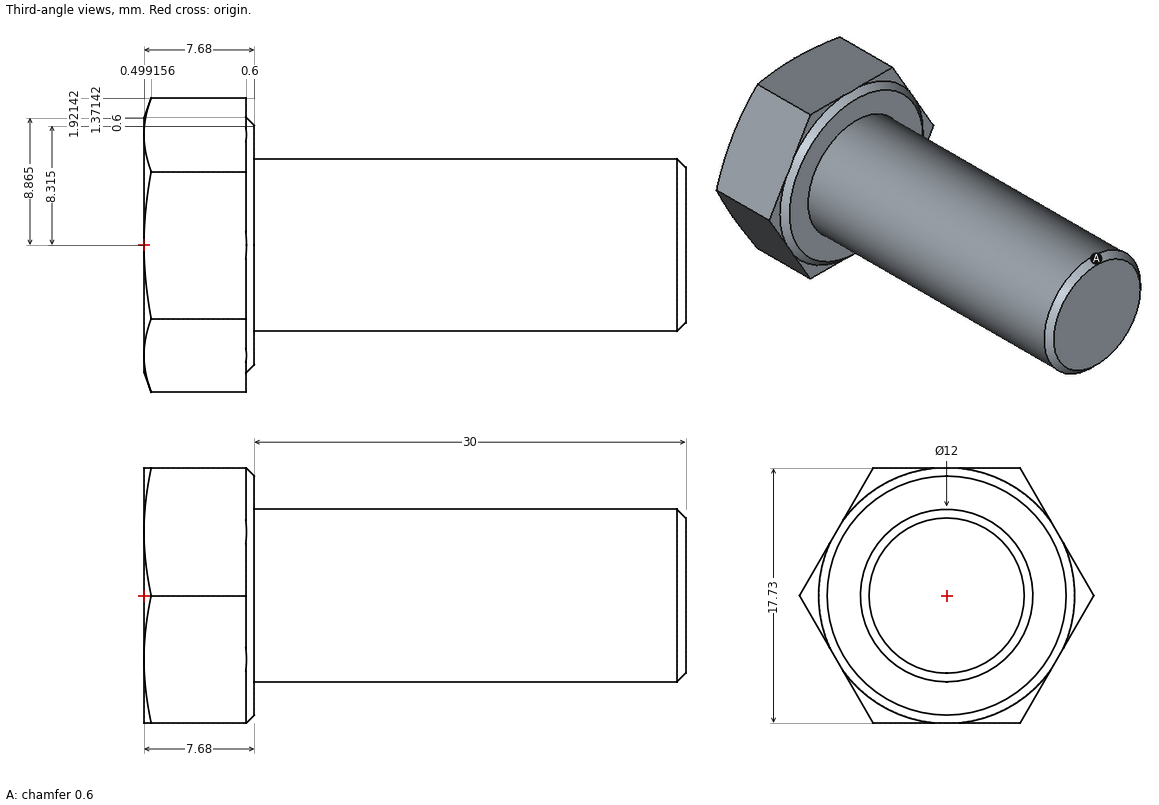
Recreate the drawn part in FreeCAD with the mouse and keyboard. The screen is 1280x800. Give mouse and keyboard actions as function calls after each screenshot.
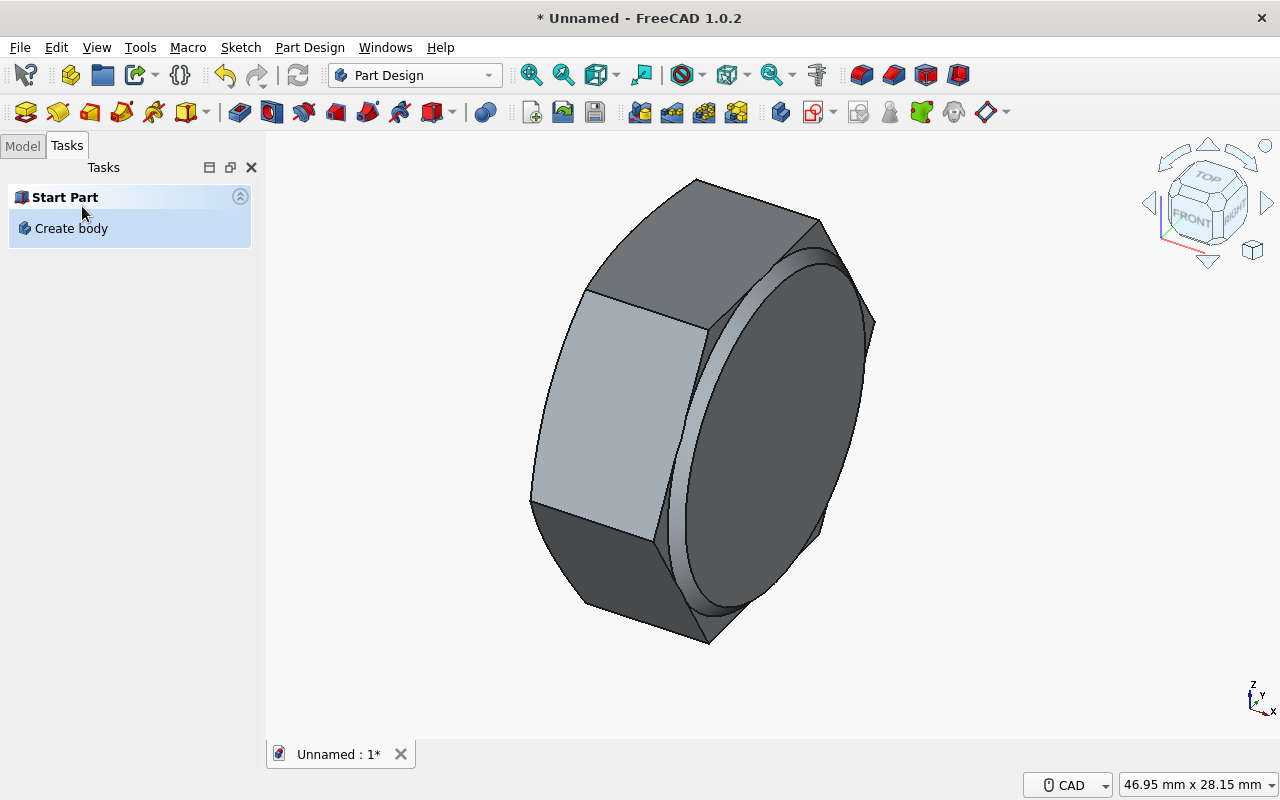
click(532, 76)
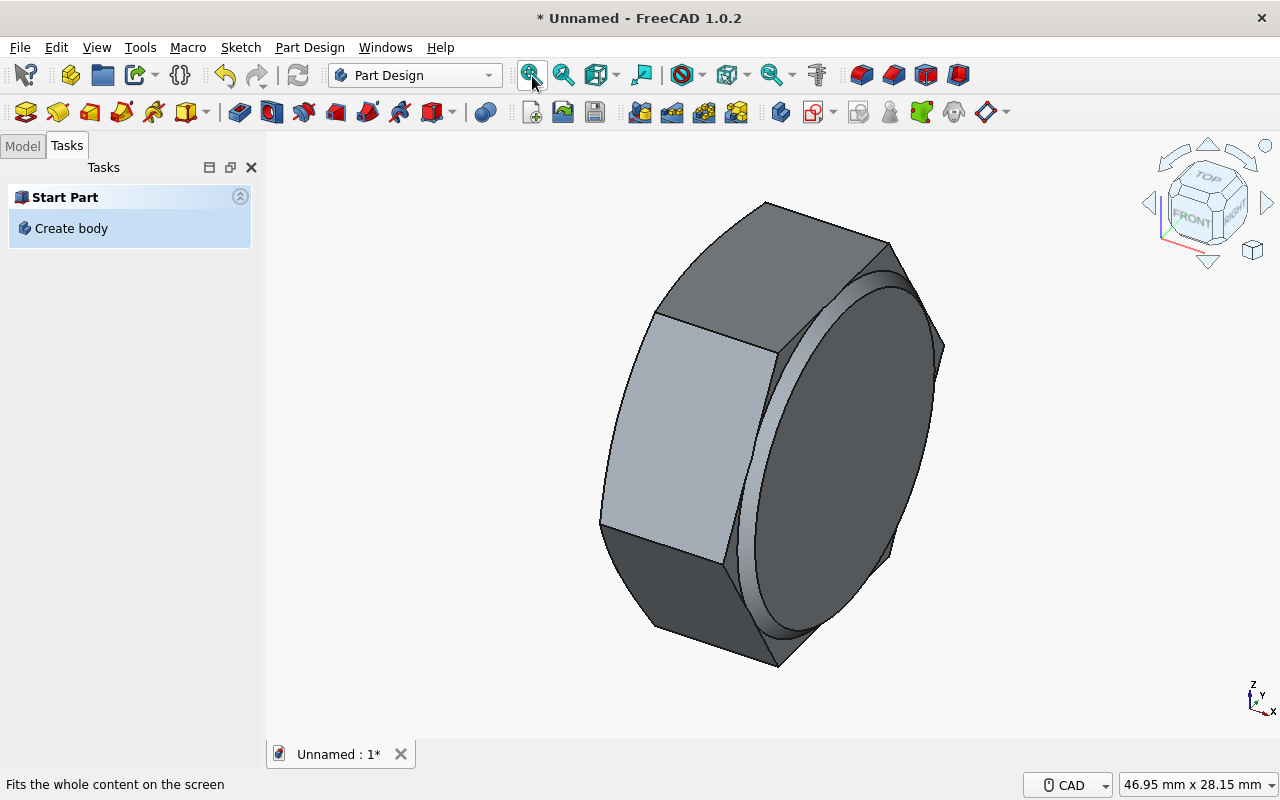
click(845, 458)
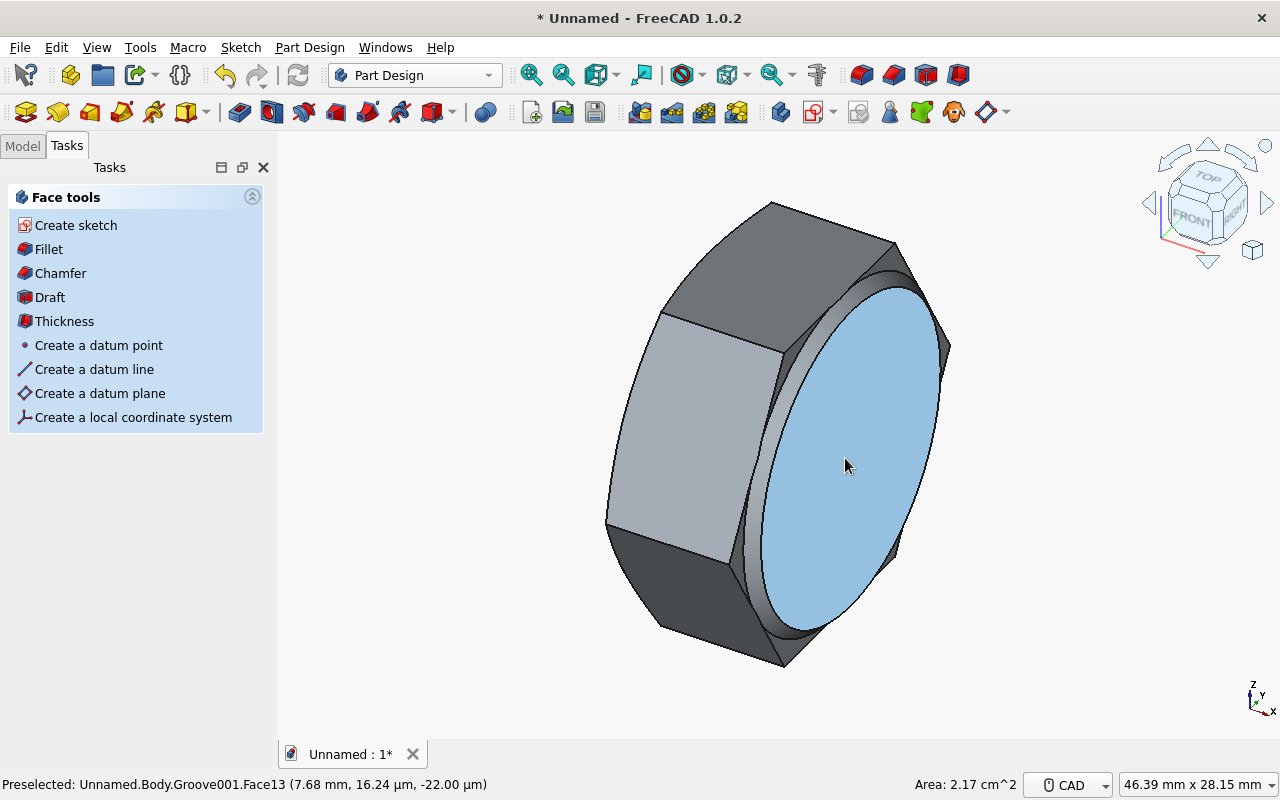
click(814, 112)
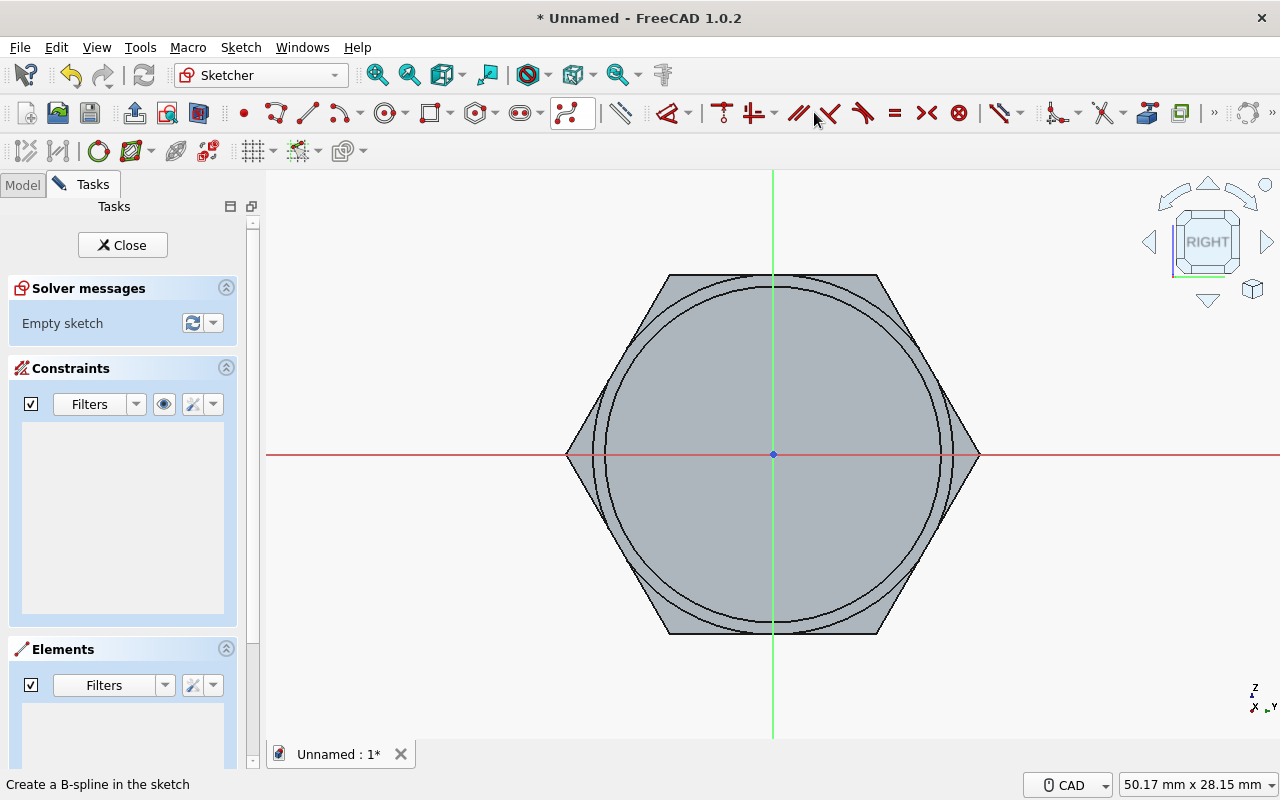
scroll(912, 454, up, 2)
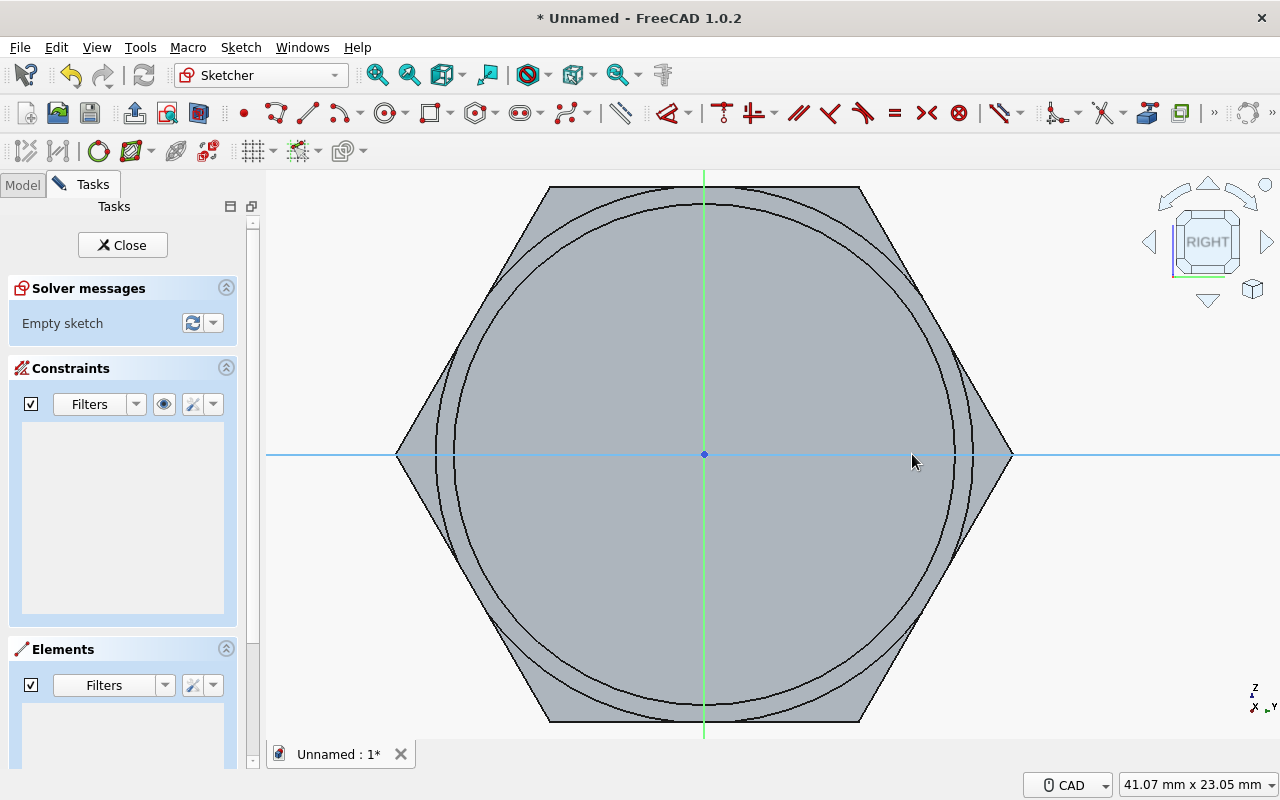
click(386, 114)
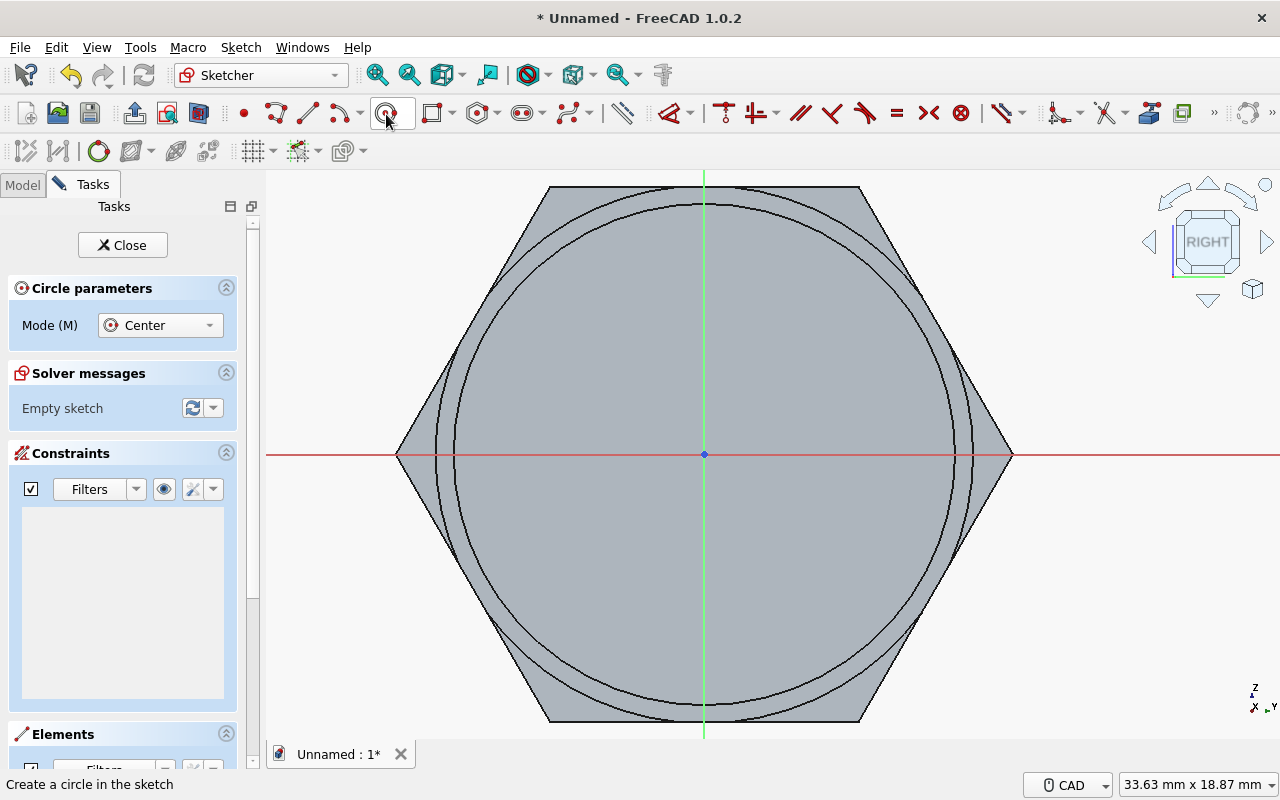
click(704, 454)
click(832, 327)
key(Escape)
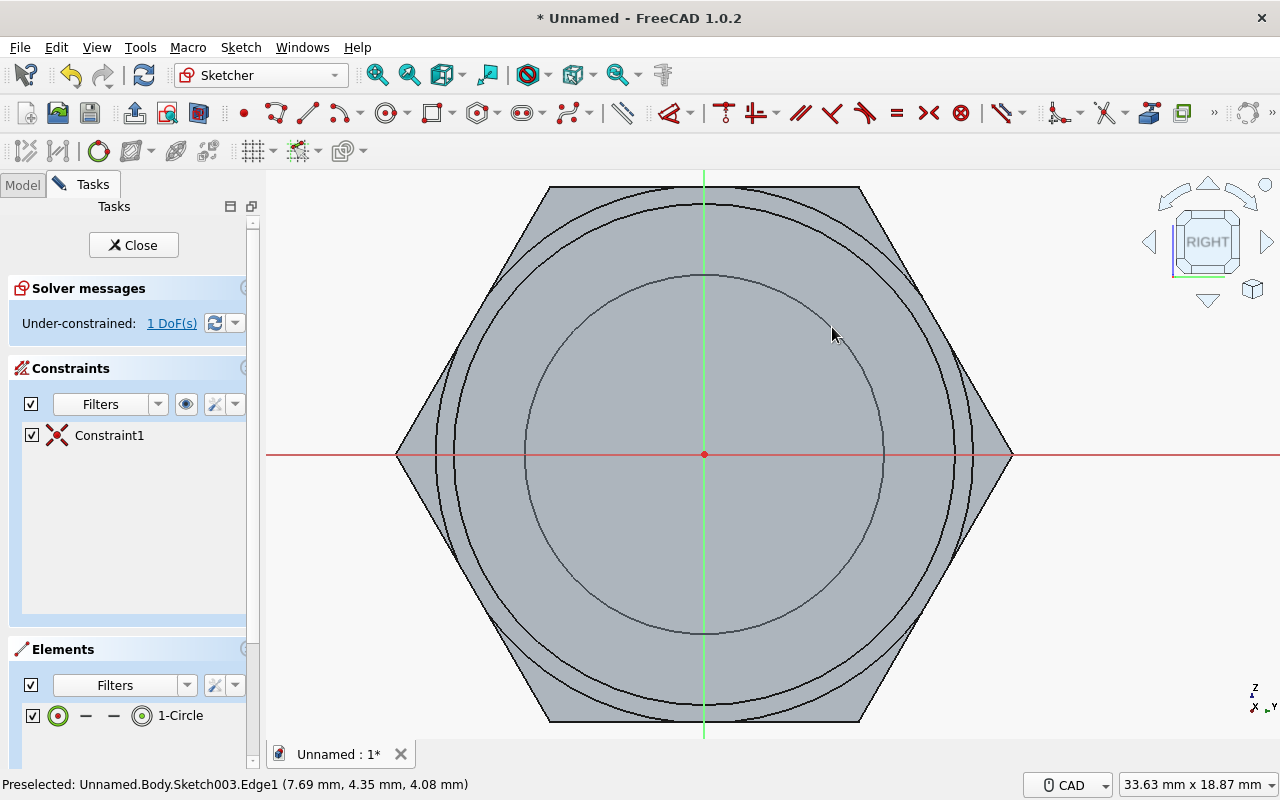
click(670, 114)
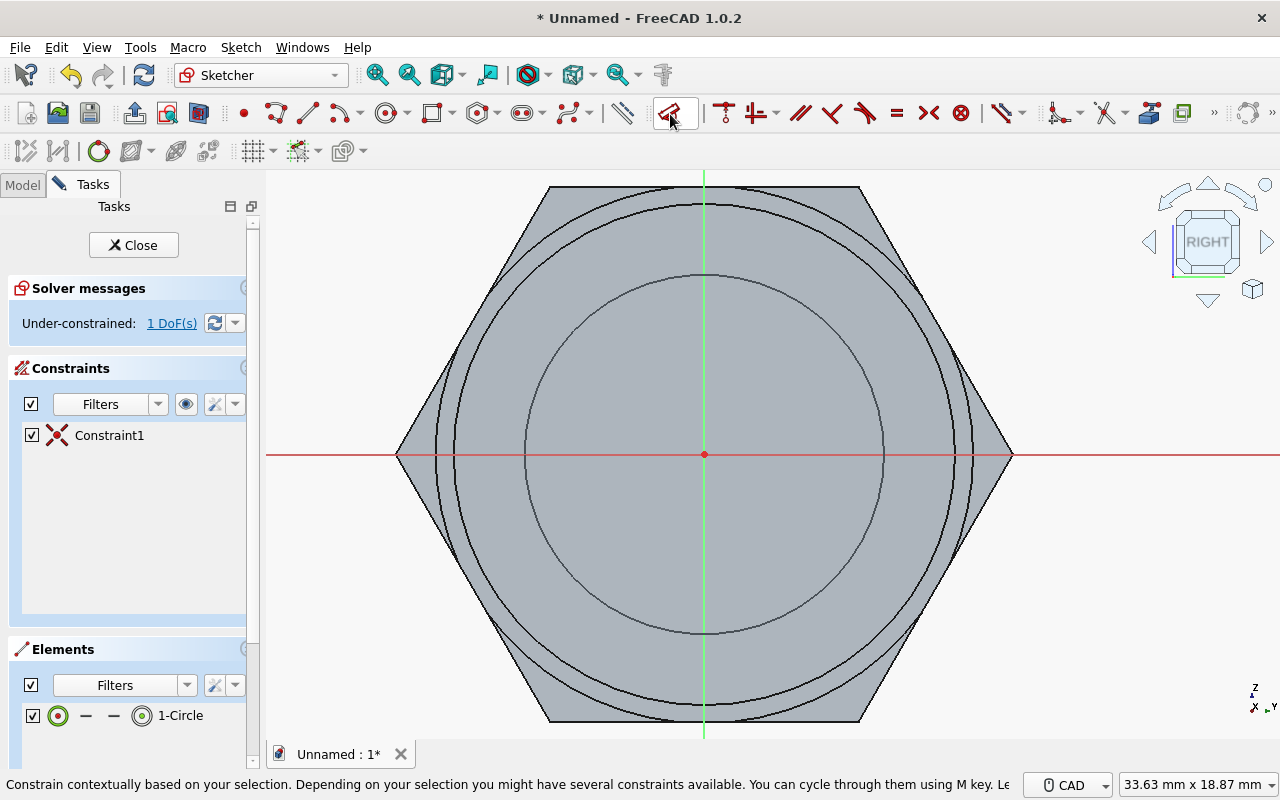
click(831, 327)
click(854, 304)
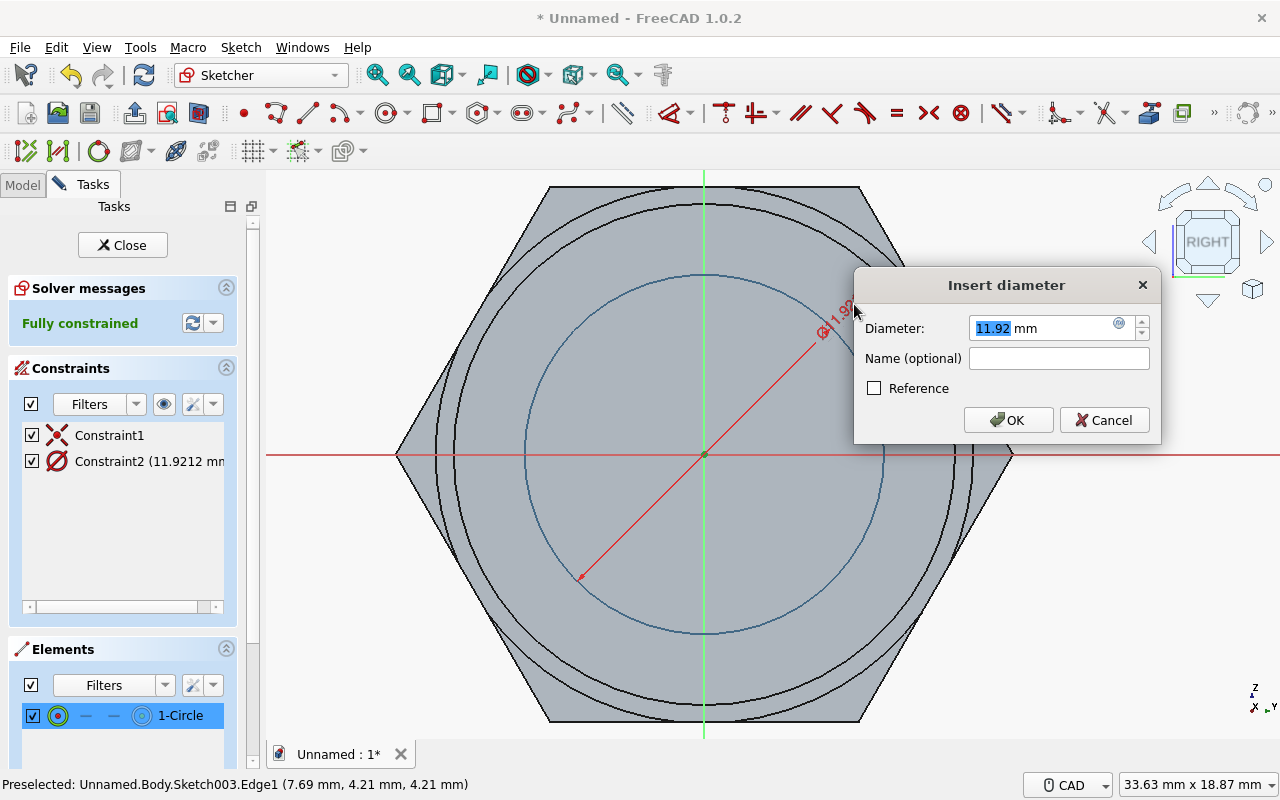
text(12)
key(Return)
key(Escape)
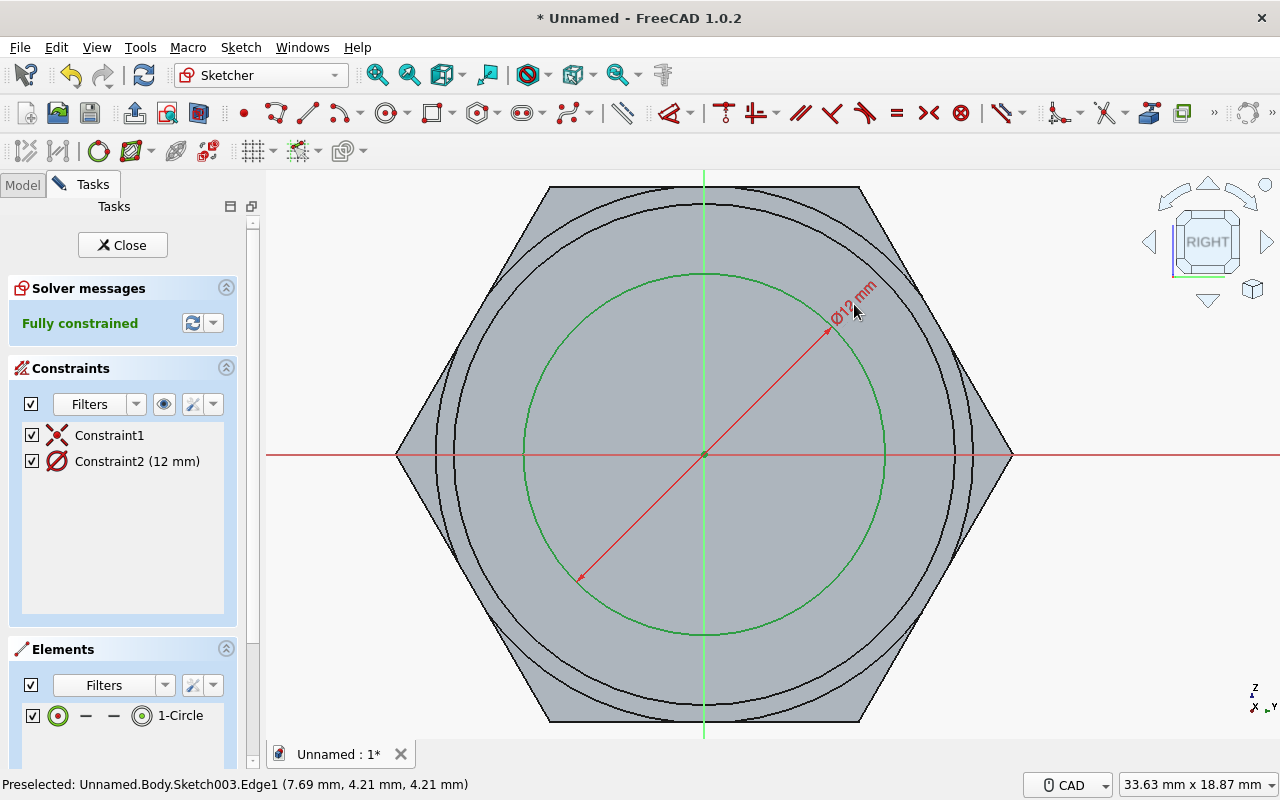
click(123, 245)